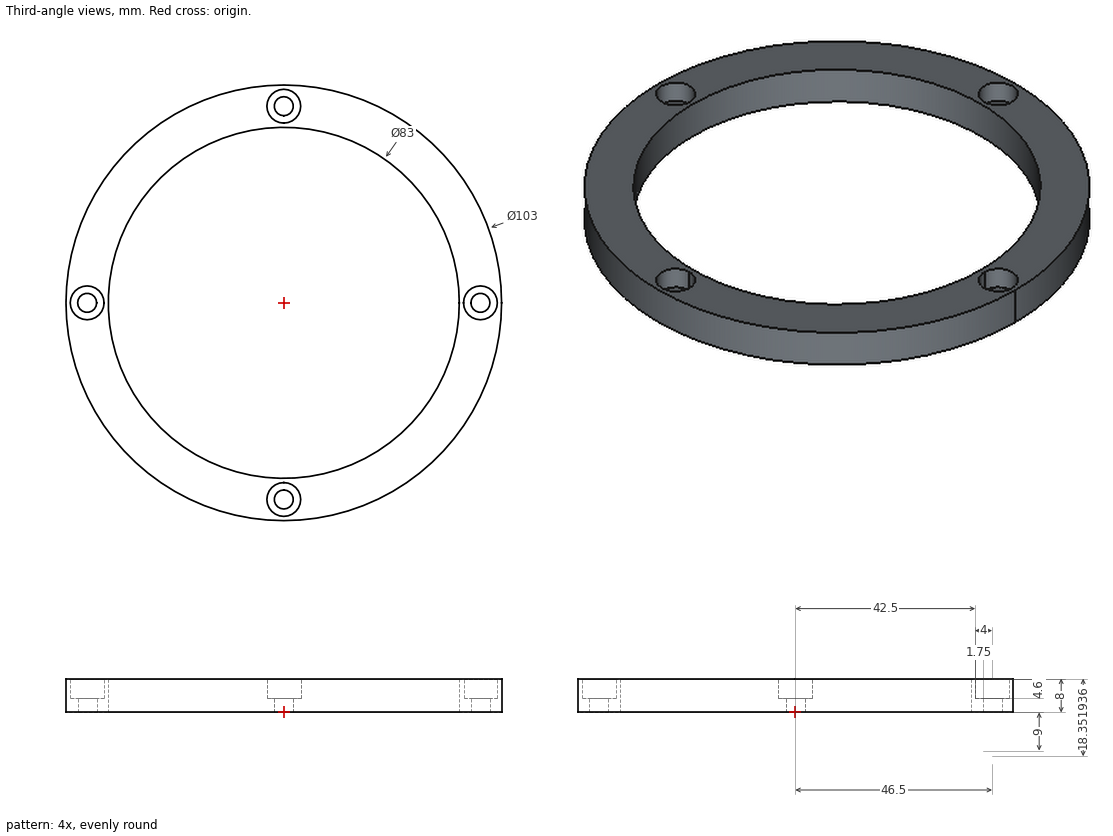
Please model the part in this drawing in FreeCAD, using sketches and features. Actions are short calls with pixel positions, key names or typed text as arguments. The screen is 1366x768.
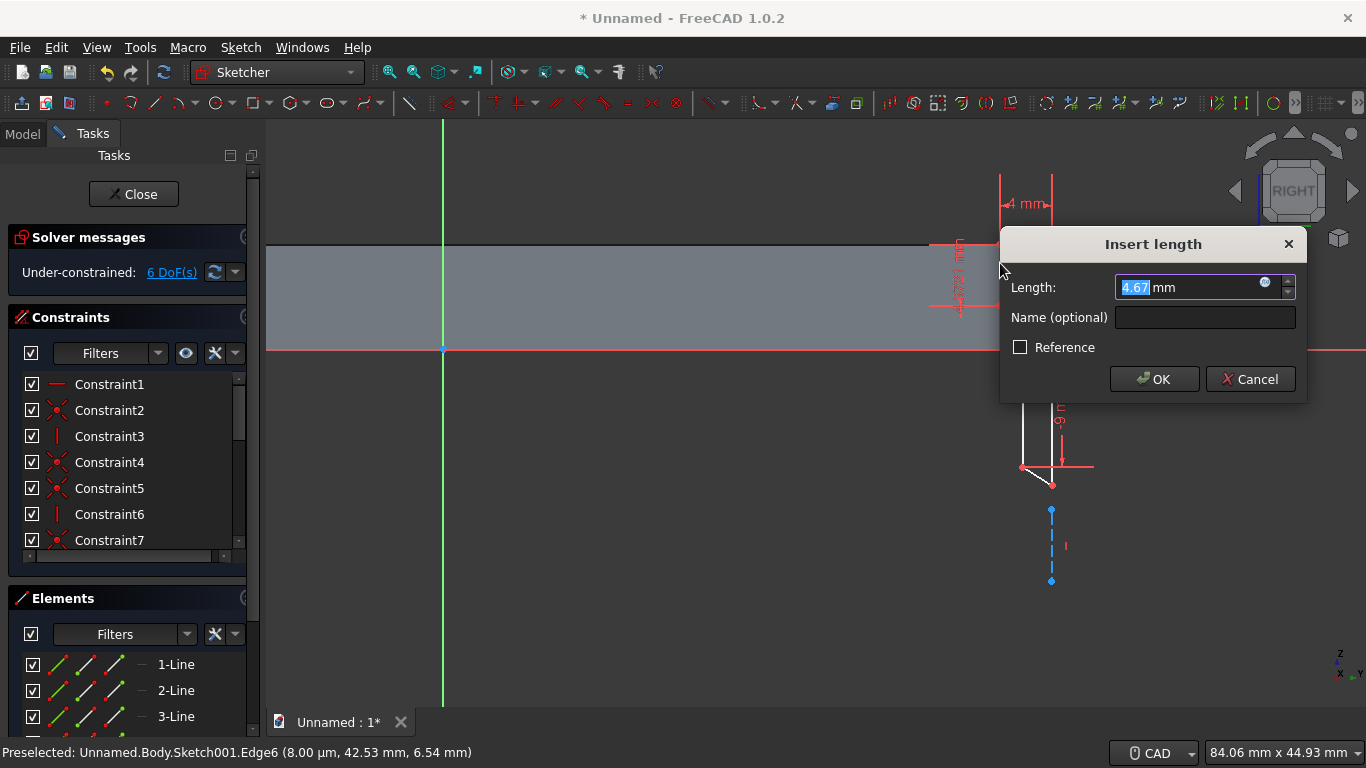
text(4.6)
key(Return)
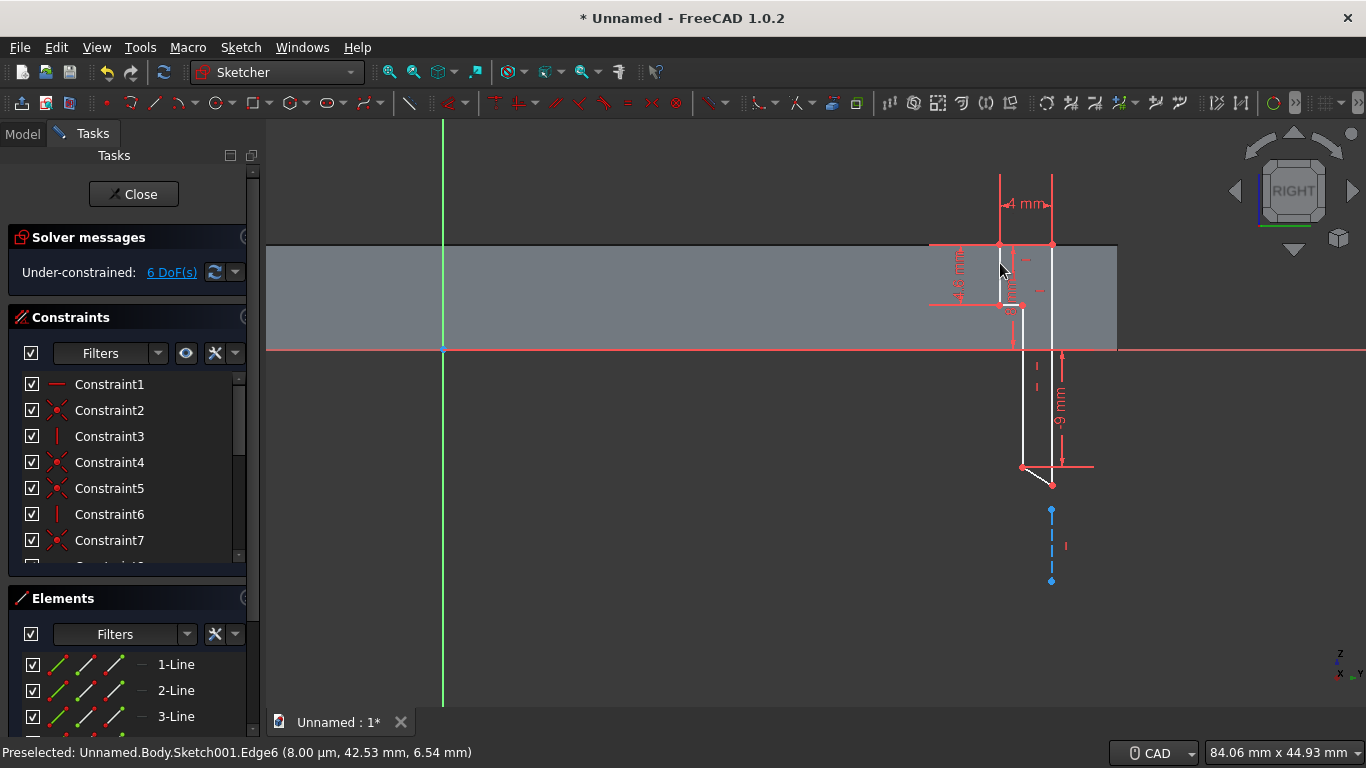
scroll(1009, 305, up, 3)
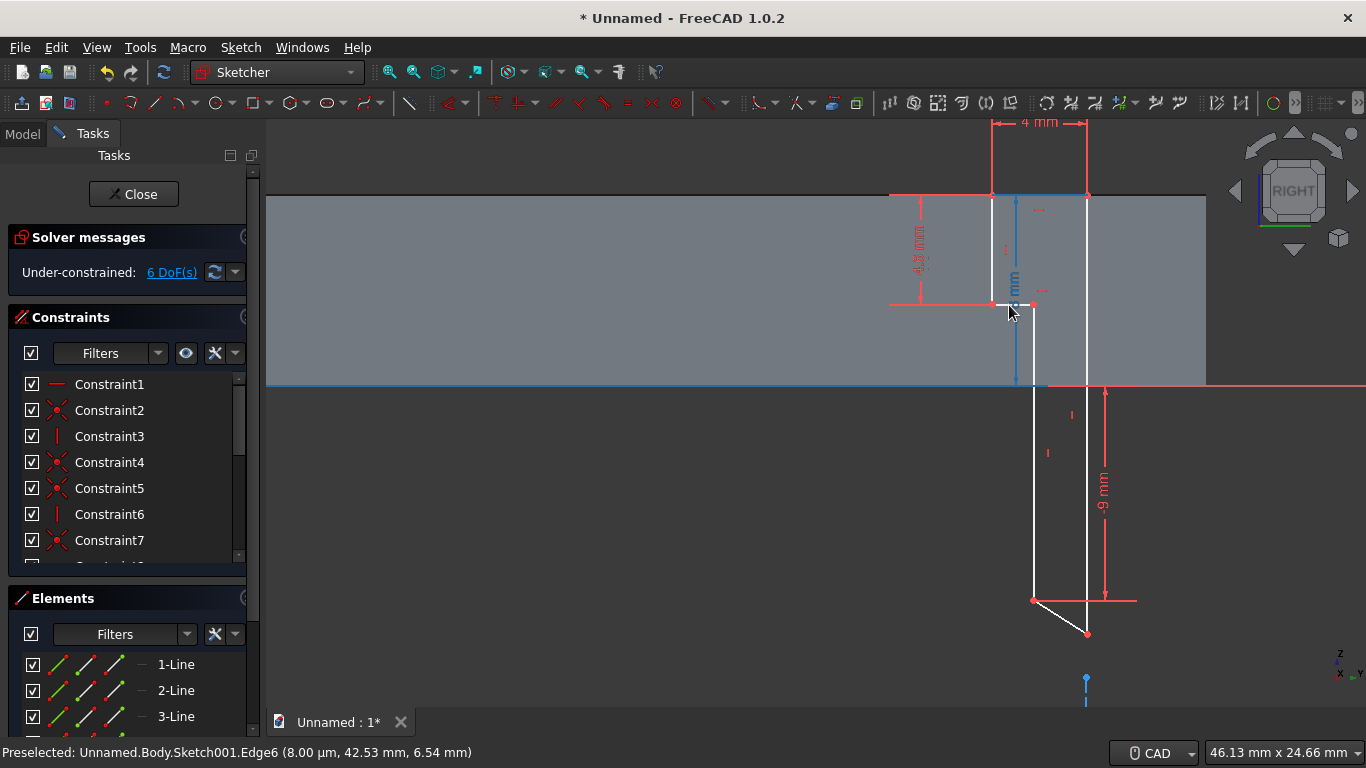
click(1005, 305)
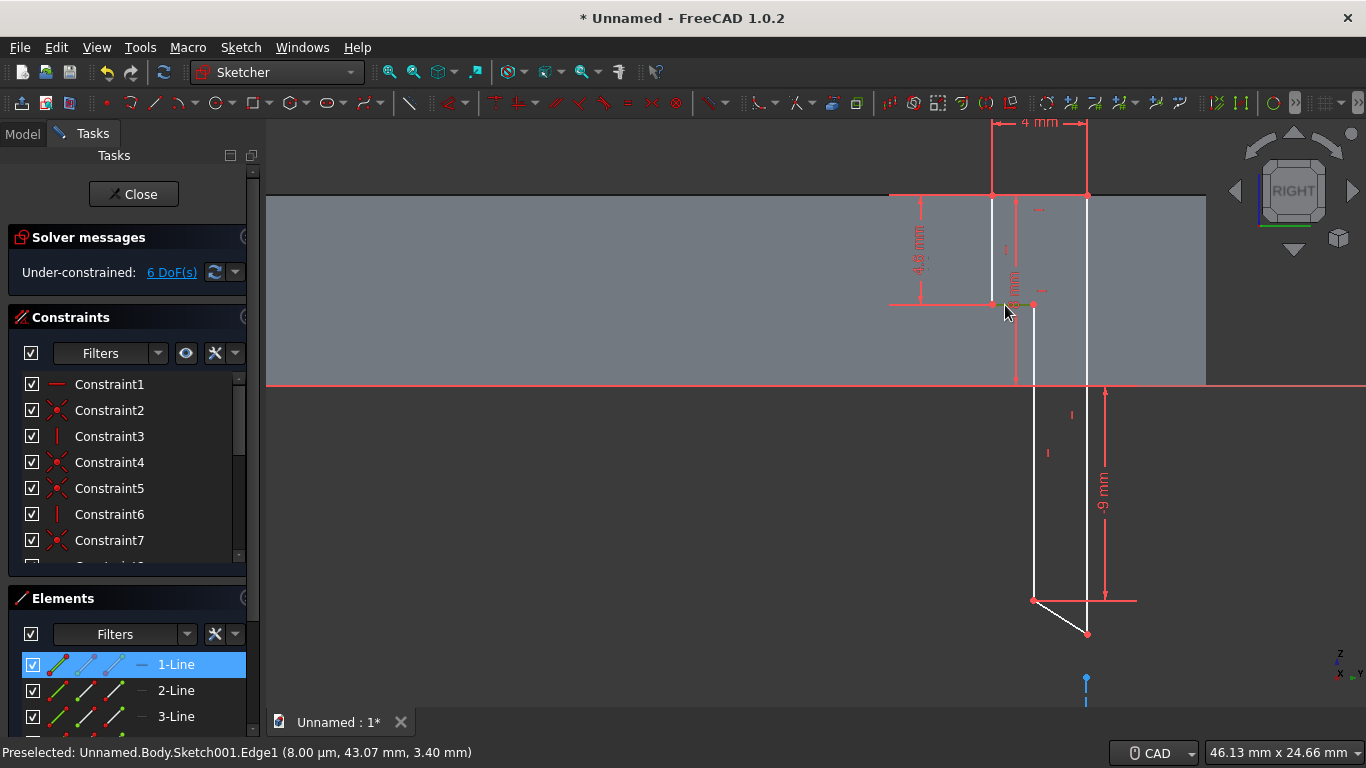
key(l)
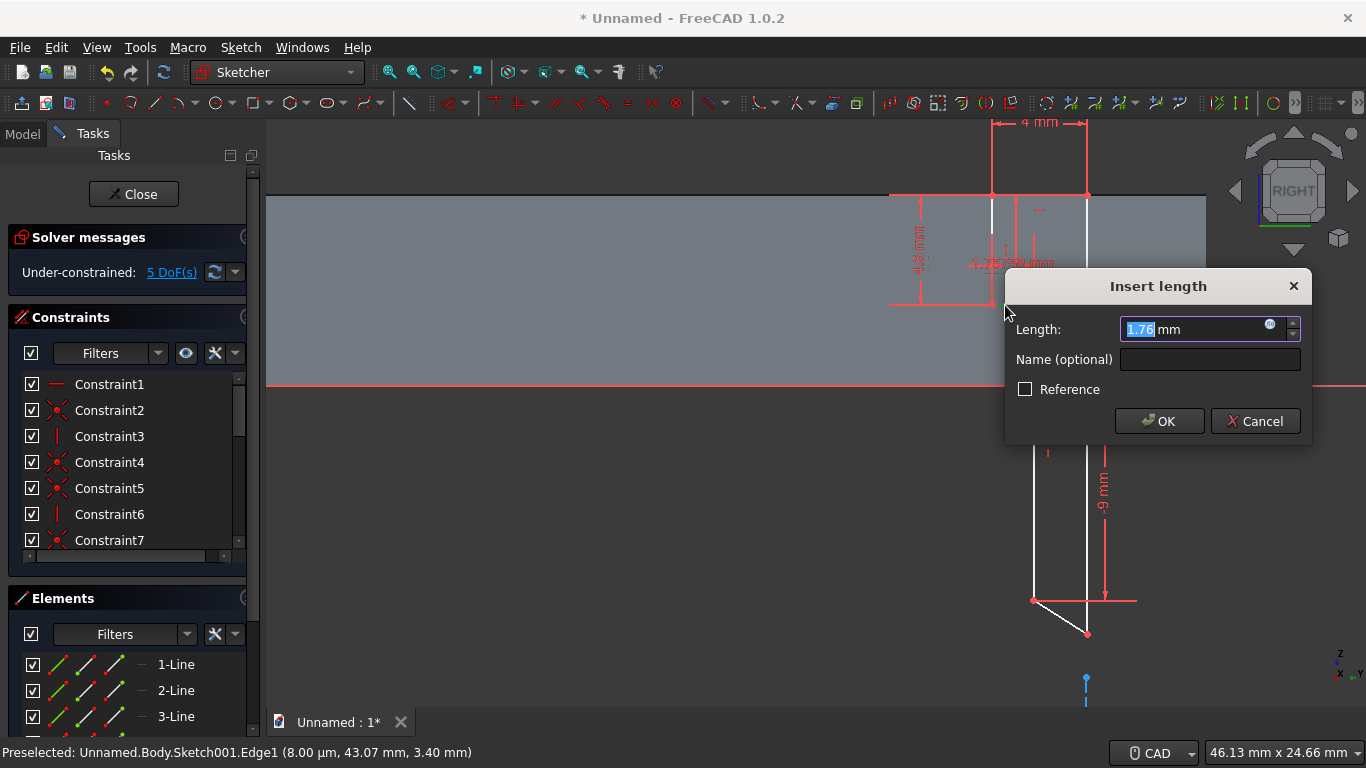
text(1.75)
key(Return)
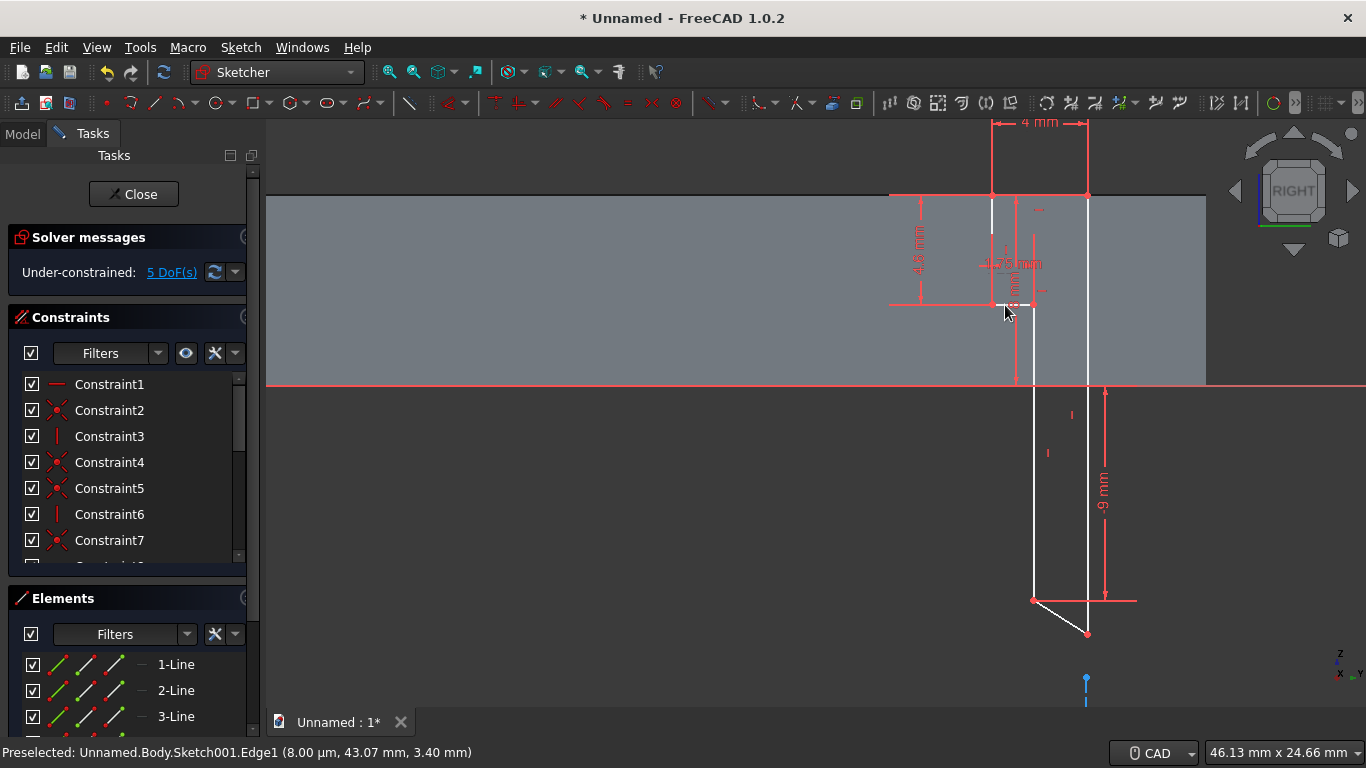
click(992, 305)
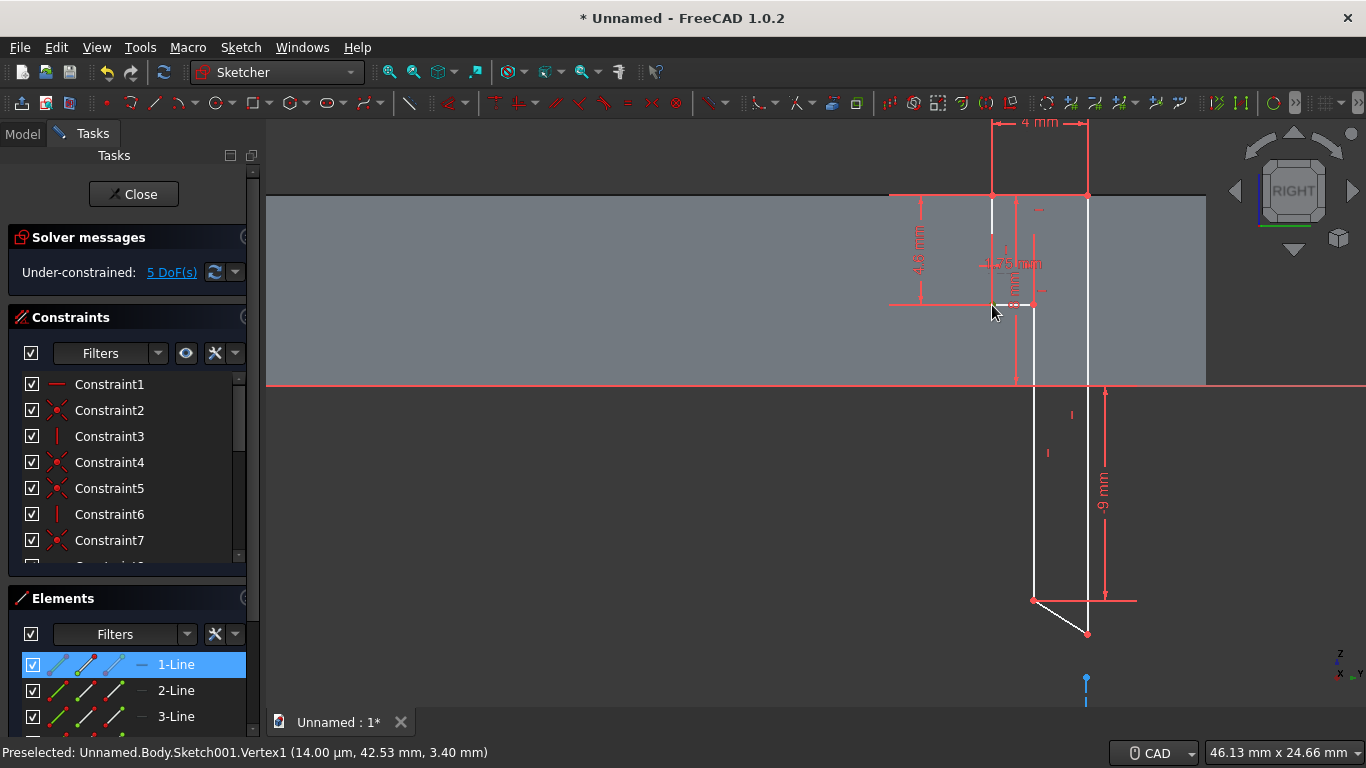
key(l)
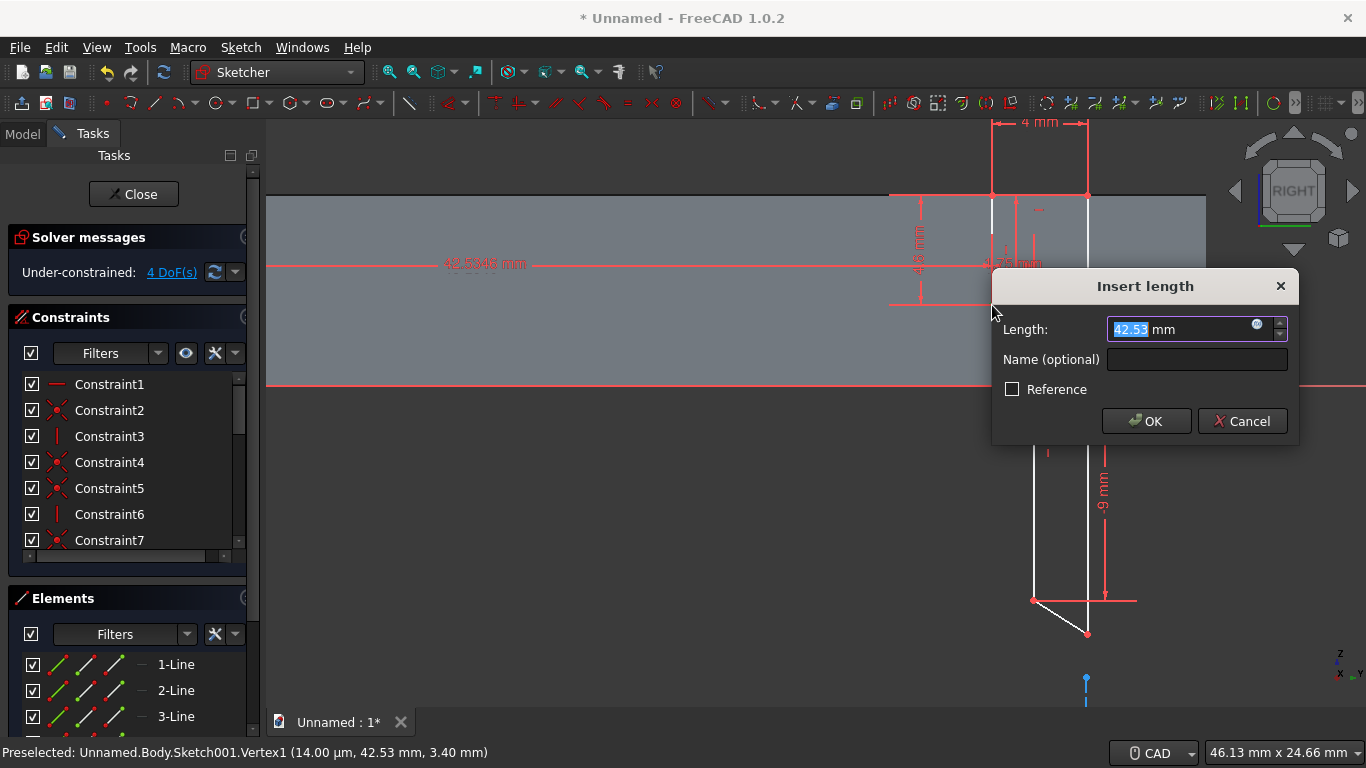
text(42.5)
key(Return)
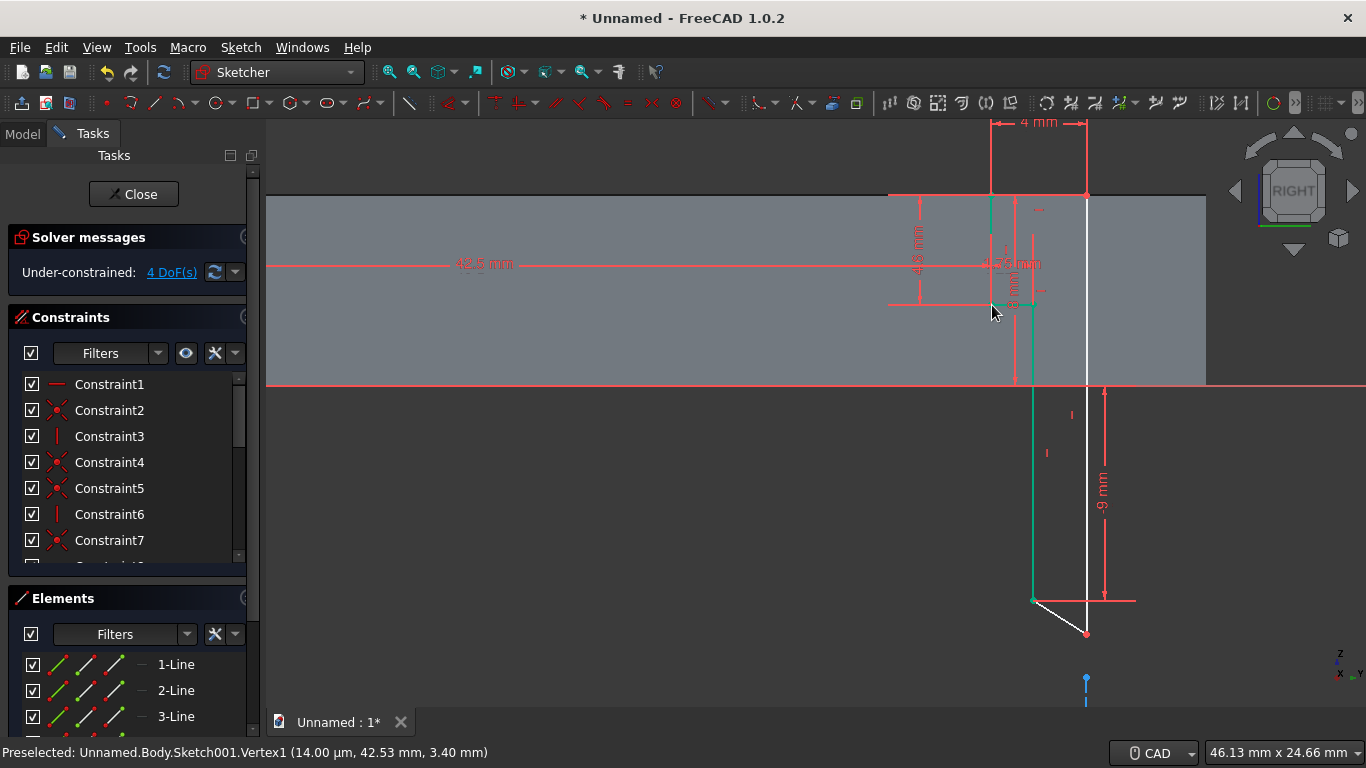
click(1086, 677)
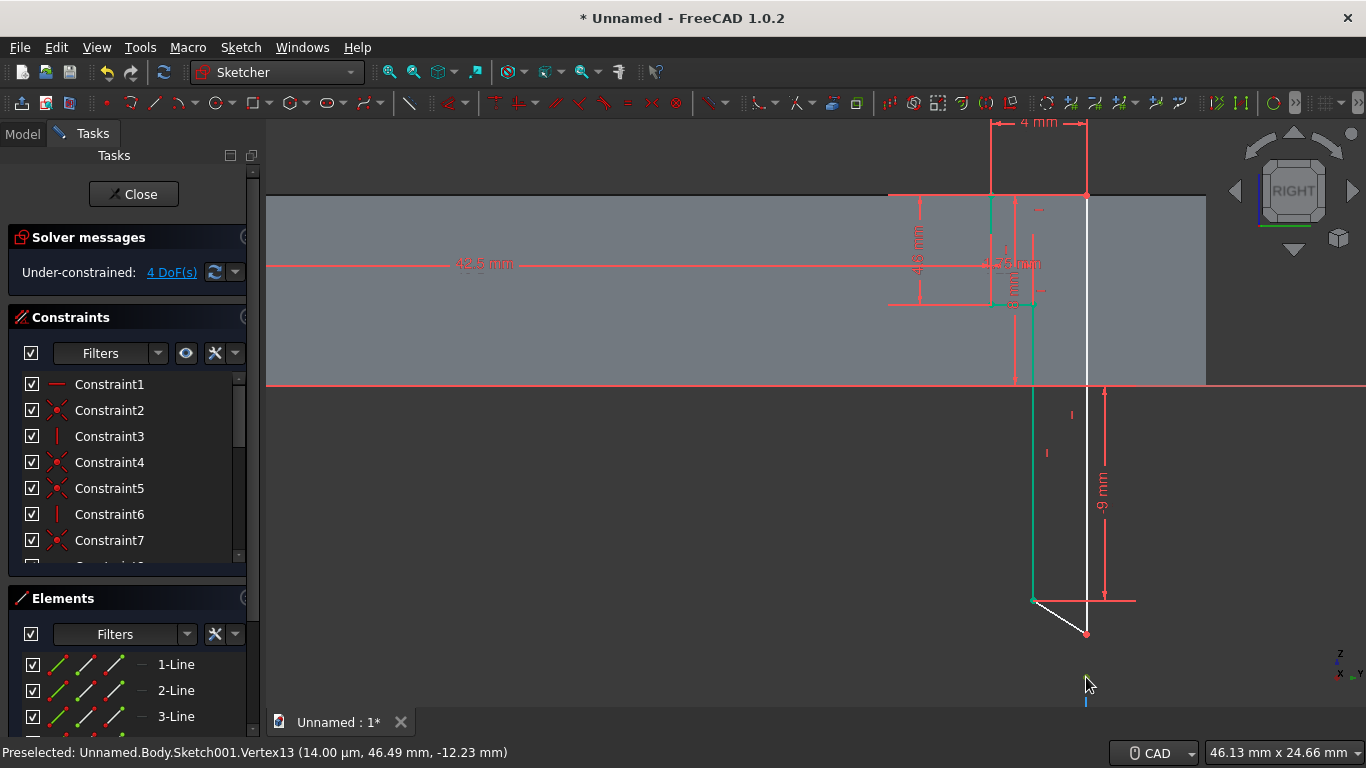
key(l)